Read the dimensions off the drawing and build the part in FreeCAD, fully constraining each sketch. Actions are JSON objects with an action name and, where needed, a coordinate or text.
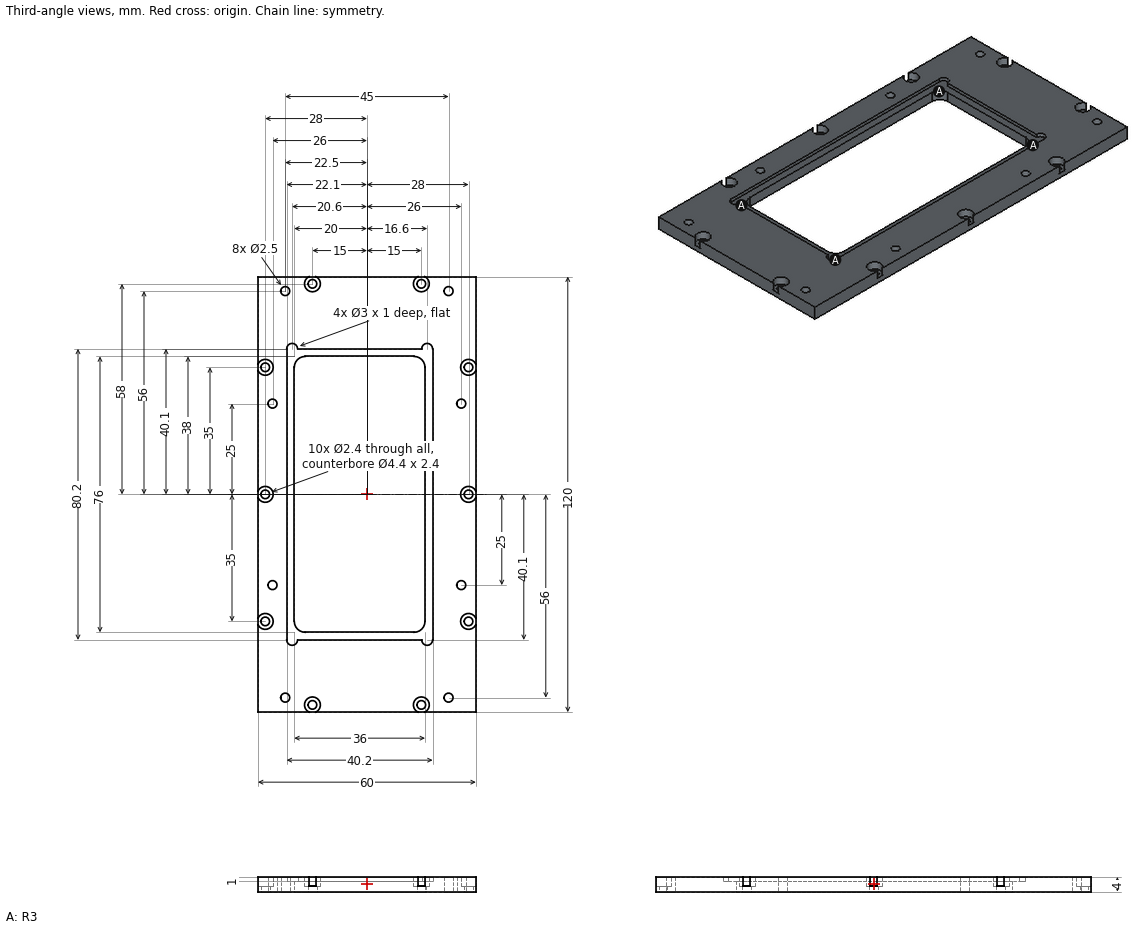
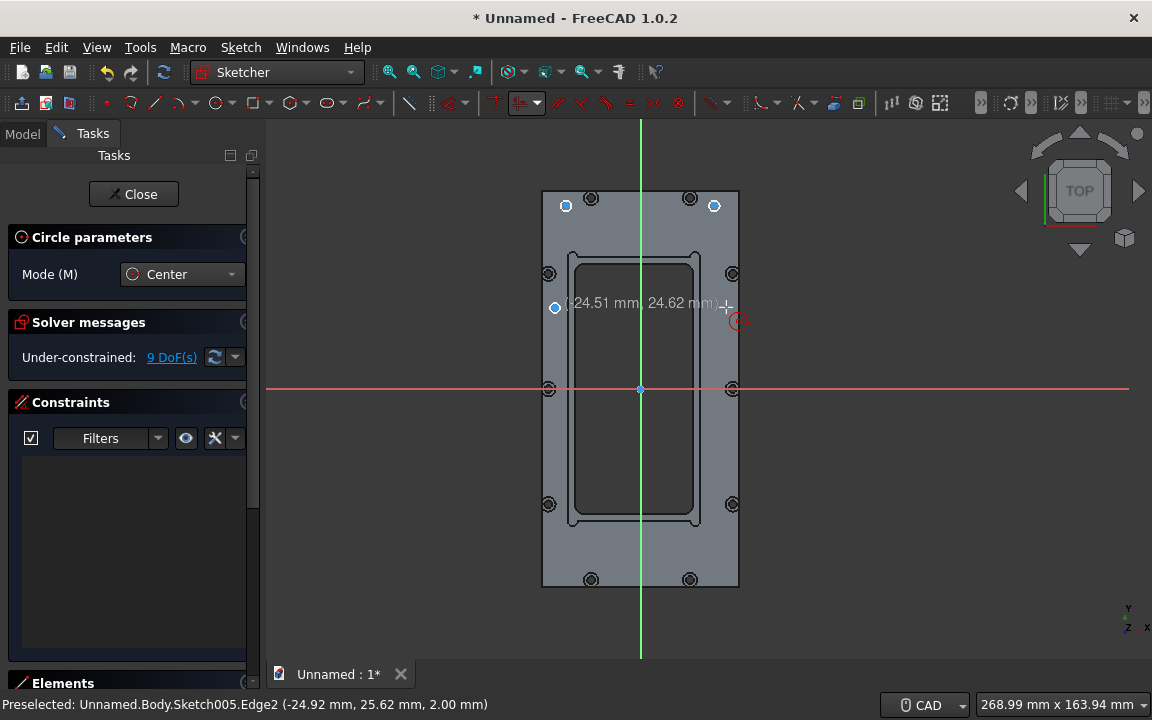
{"action": "left_click", "coordinate": [726, 307]}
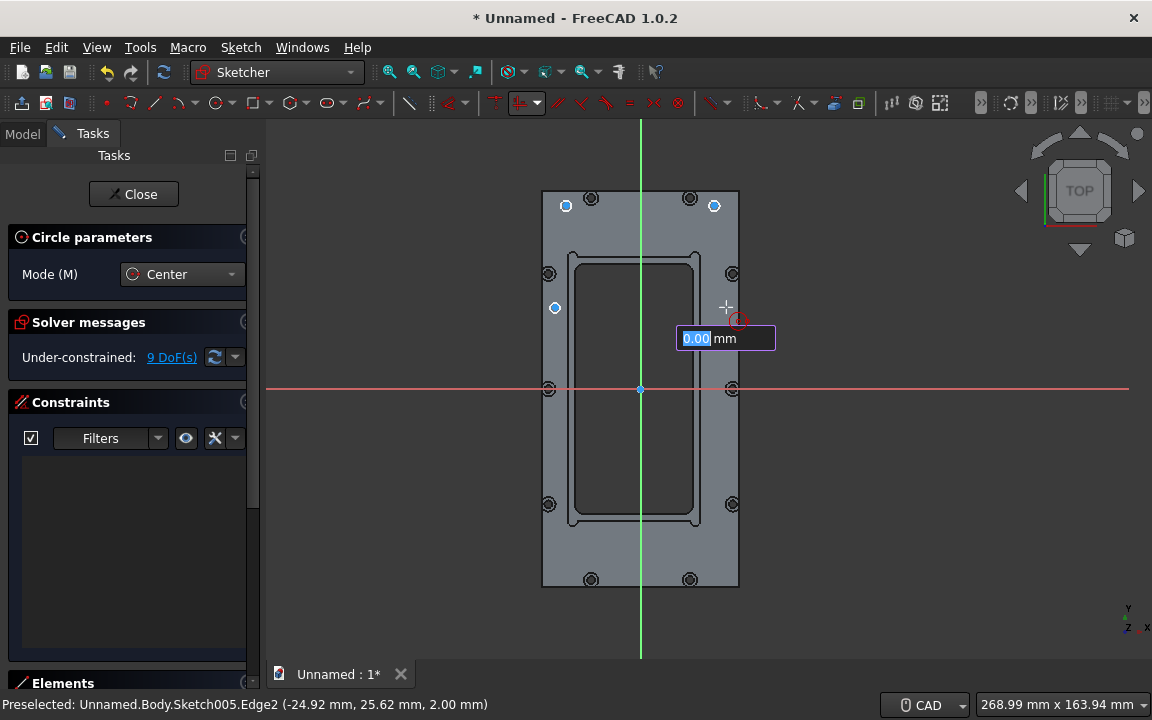
{"action": "scroll", "coordinate": [729, 304], "scroll_direction": "up", "scroll_amount": 7}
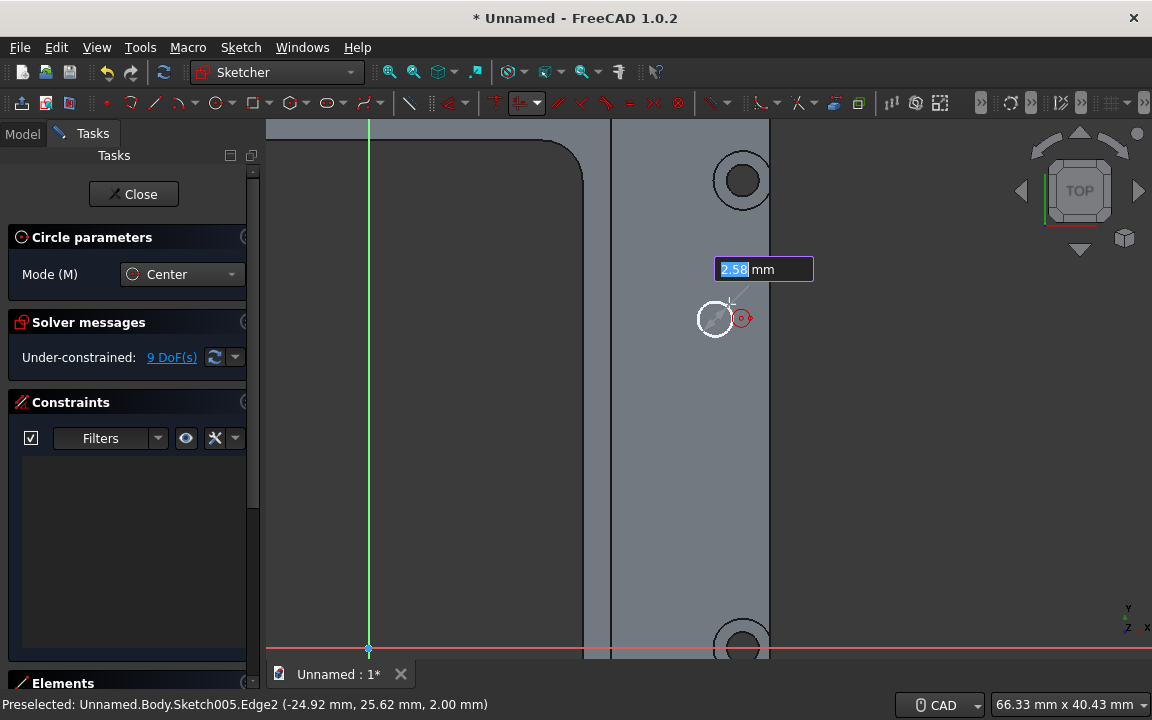
{"action": "left_click", "coordinate": [728, 302]}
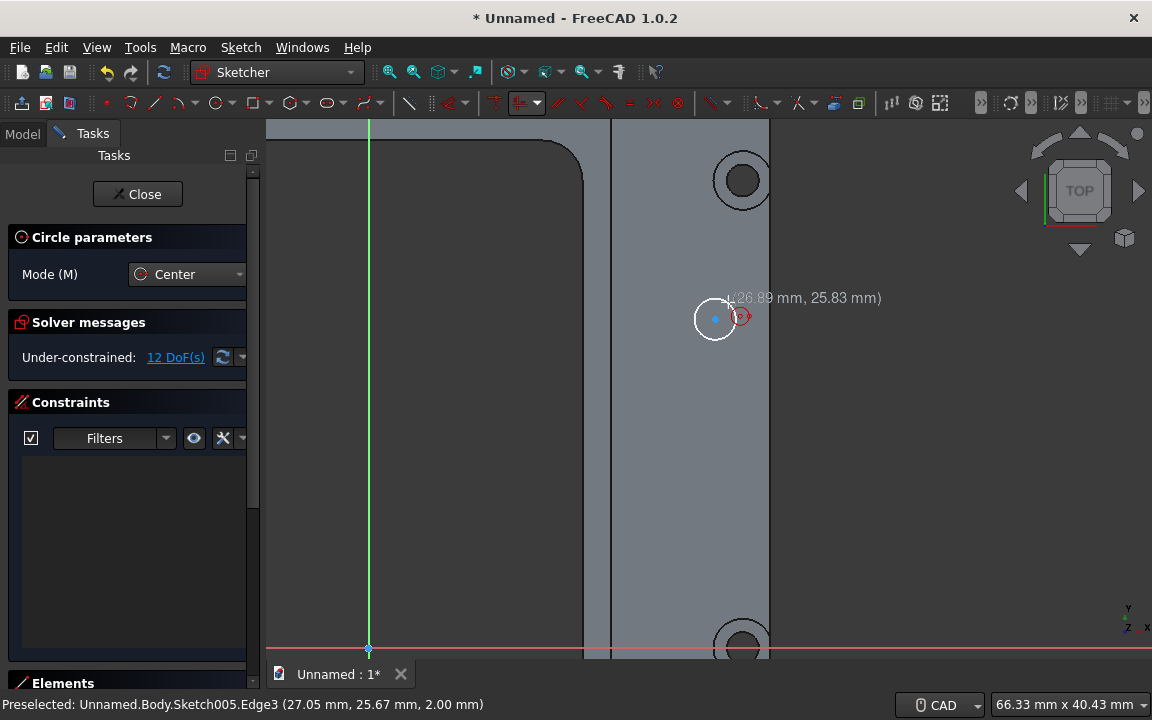
{"action": "scroll", "coordinate": [729, 304], "scroll_direction": "down", "scroll_amount": 7}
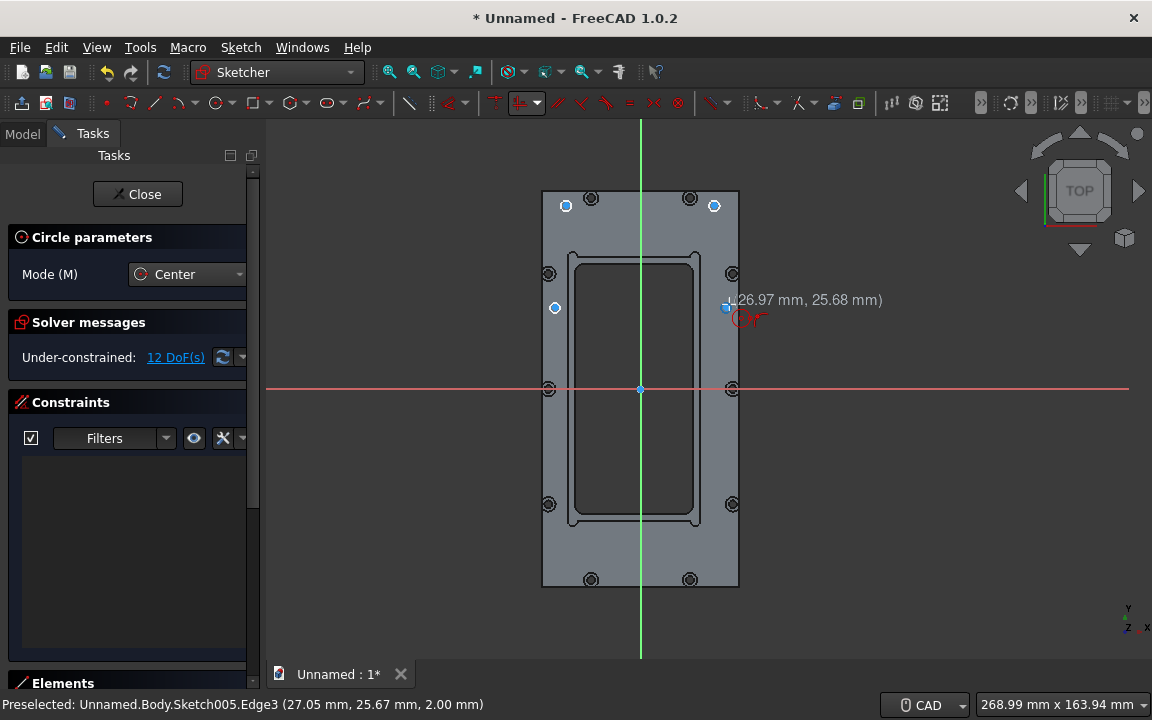
{"action": "scroll", "coordinate": [726, 471], "scroll_direction": "up", "scroll_amount": 9}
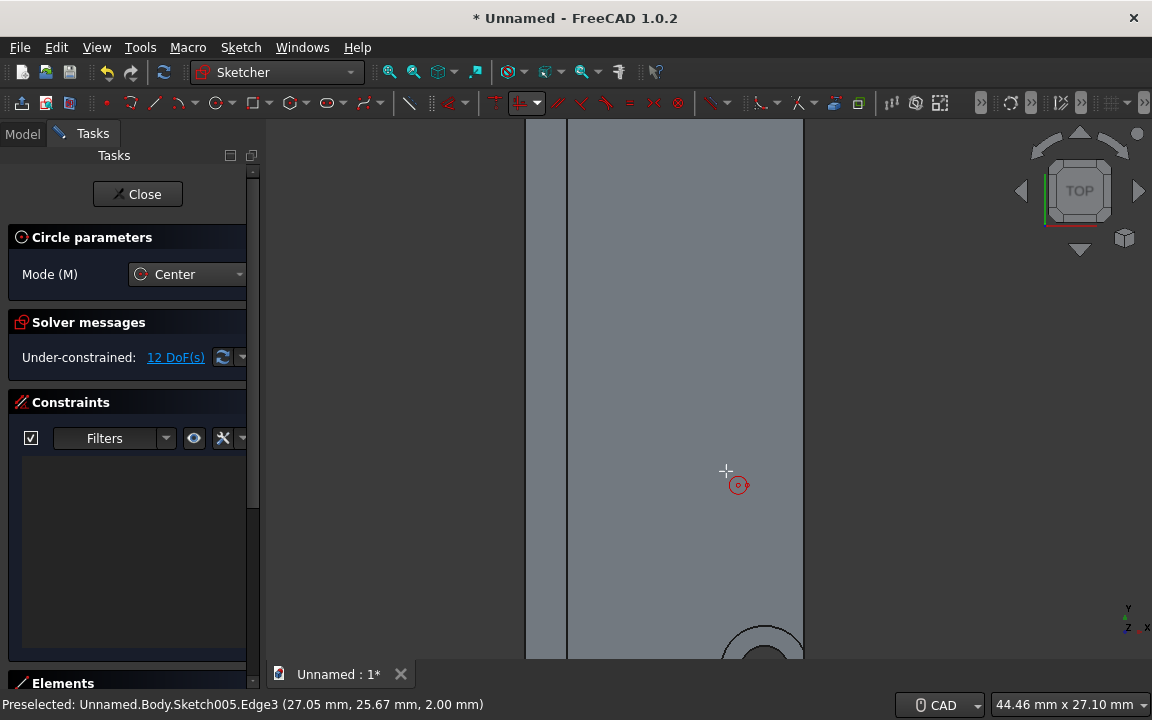
{"action": "scroll", "coordinate": [726, 472], "scroll_direction": "down", "scroll_amount": 9}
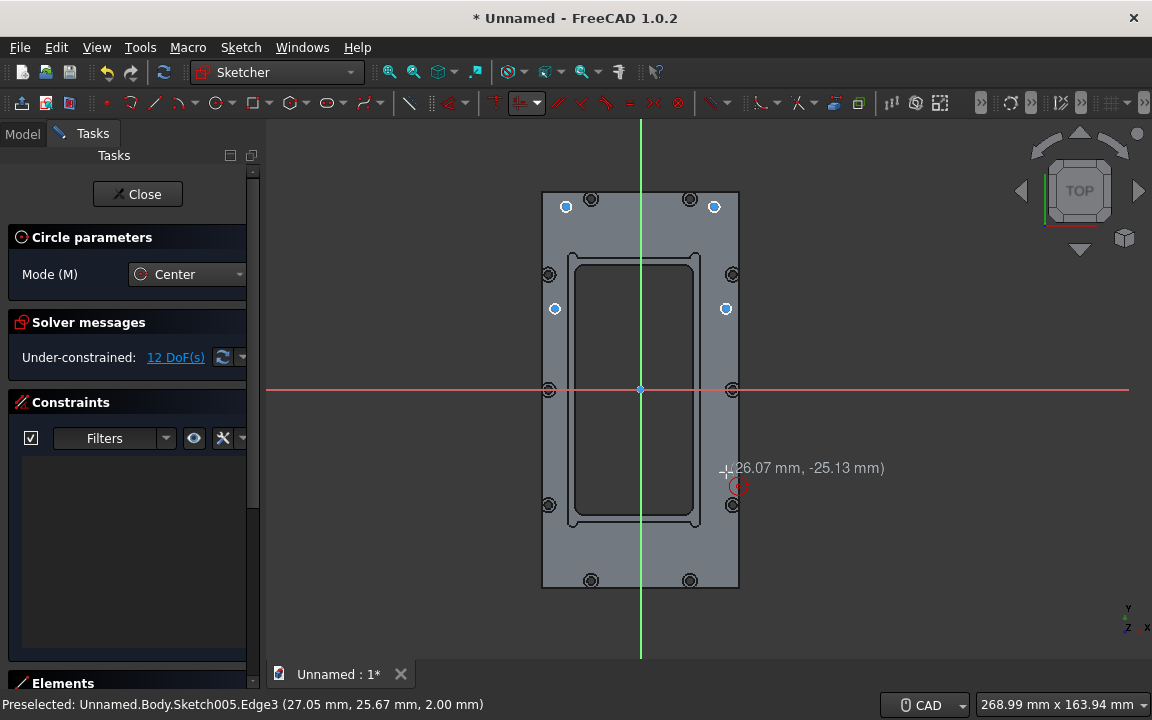
{"action": "left_click", "coordinate": [726, 472]}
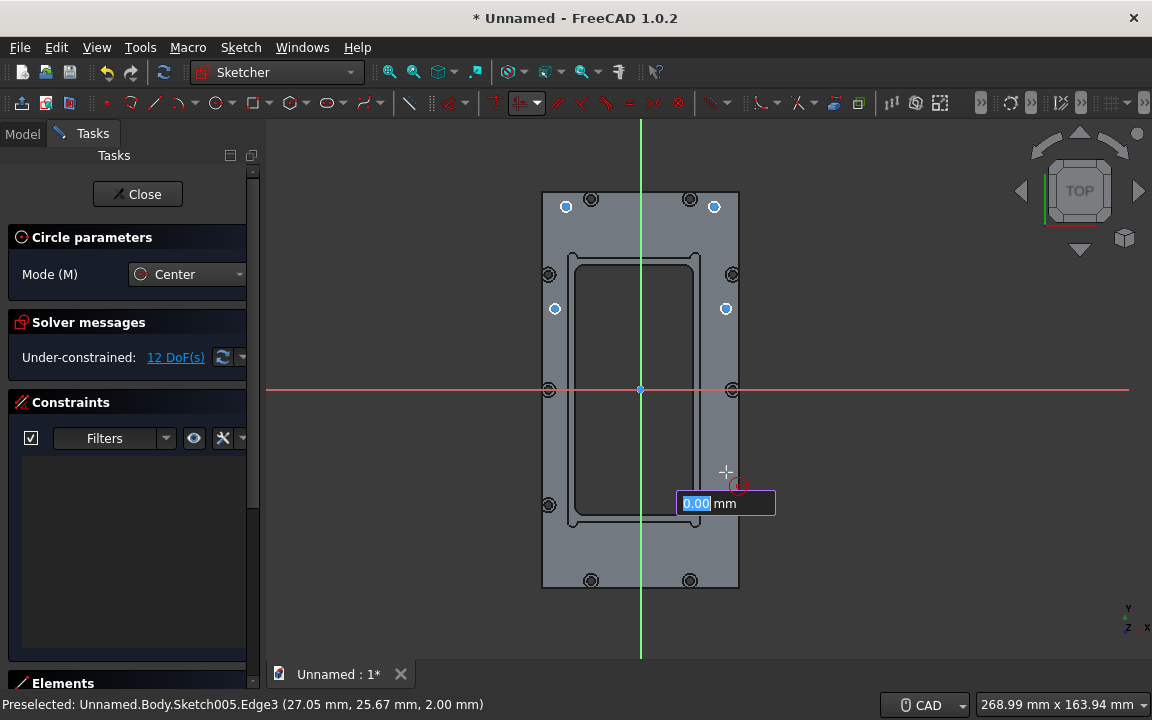
{"action": "scroll", "coordinate": [729, 469], "scroll_direction": "up", "scroll_amount": 7}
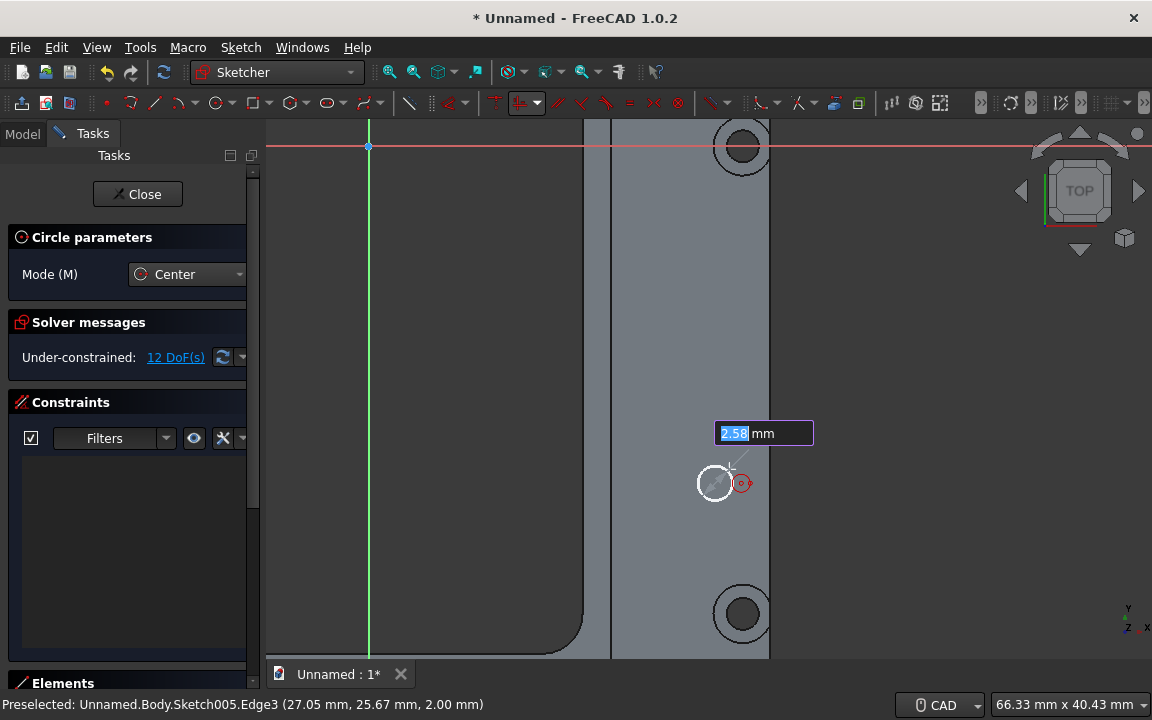
{"action": "left_click", "coordinate": [728, 468]}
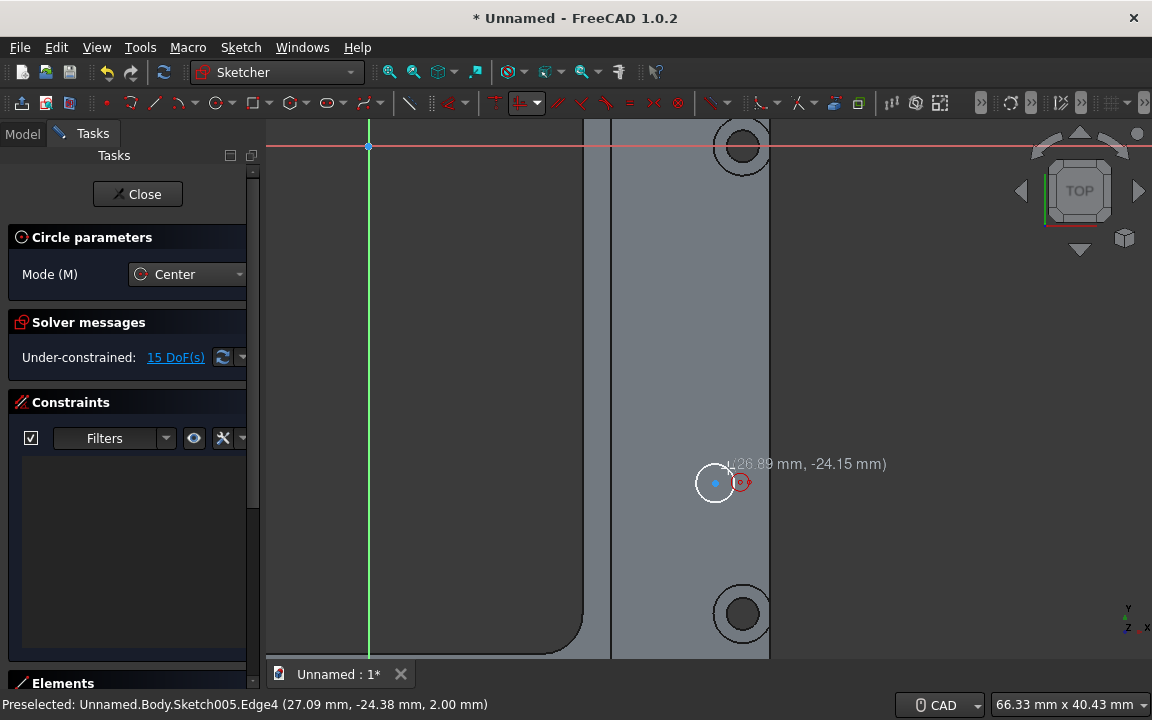
{"action": "scroll", "coordinate": [729, 468], "scroll_direction": "down", "scroll_amount": 7}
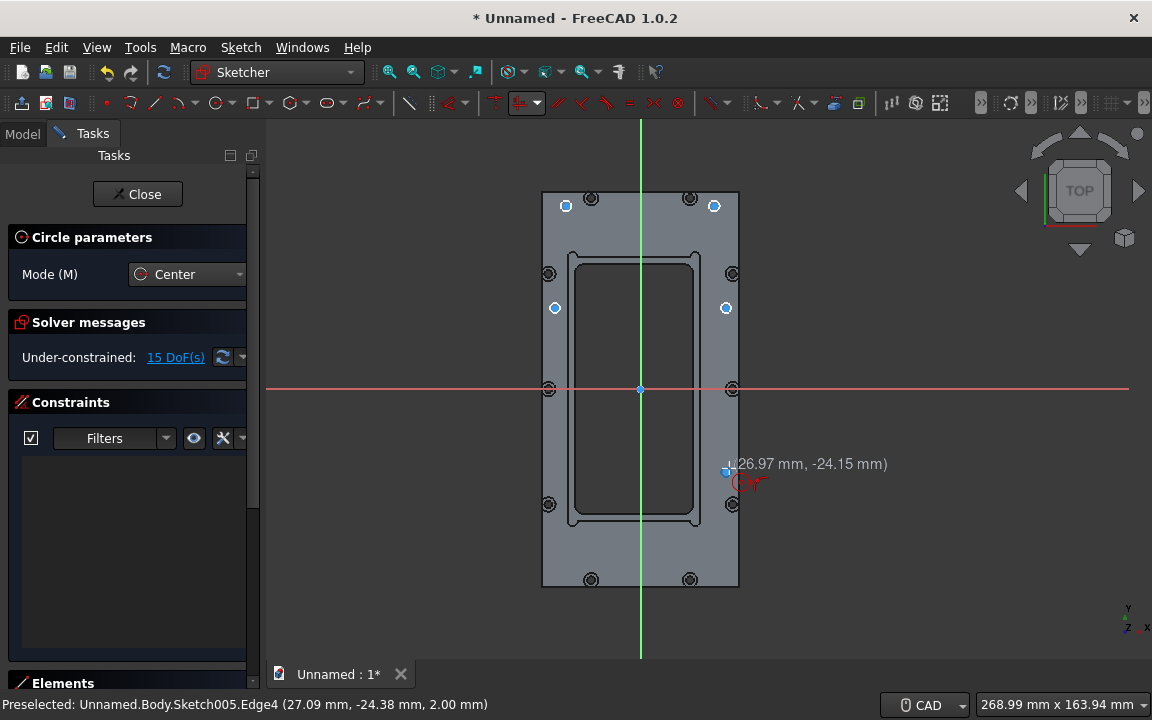
{"action": "scroll", "coordinate": [555, 472], "scroll_direction": "up", "scroll_amount": 9}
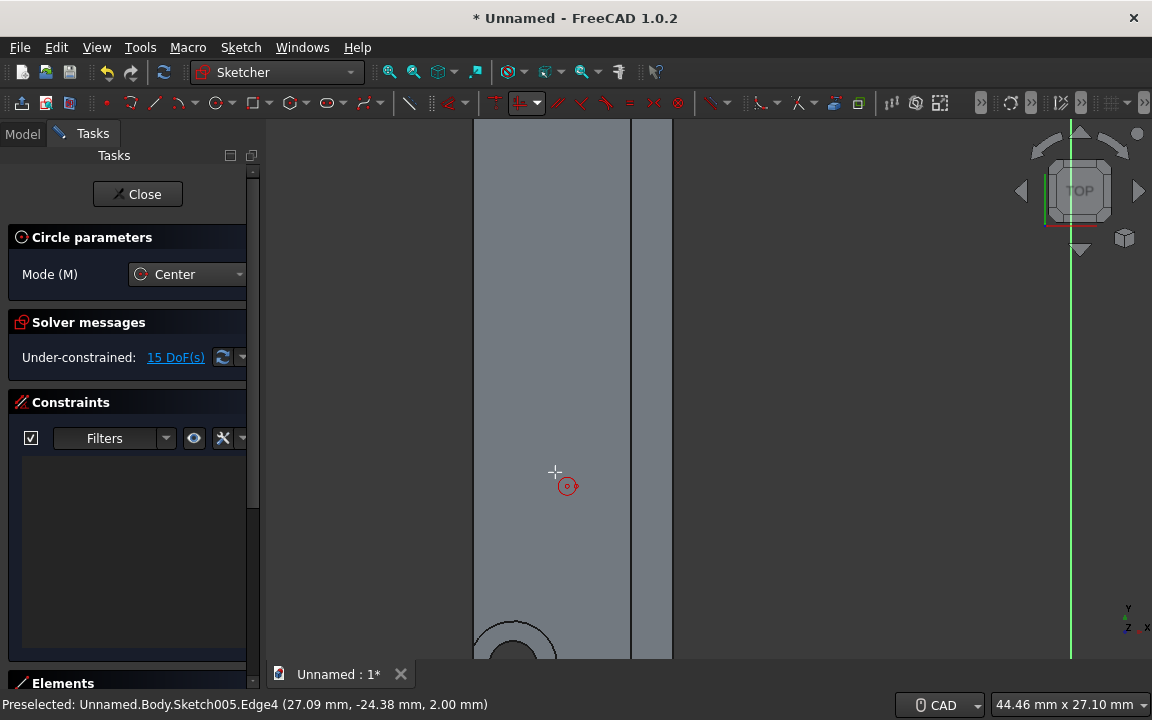
{"action": "scroll", "coordinate": [555, 472], "scroll_direction": "down", "scroll_amount": 9}